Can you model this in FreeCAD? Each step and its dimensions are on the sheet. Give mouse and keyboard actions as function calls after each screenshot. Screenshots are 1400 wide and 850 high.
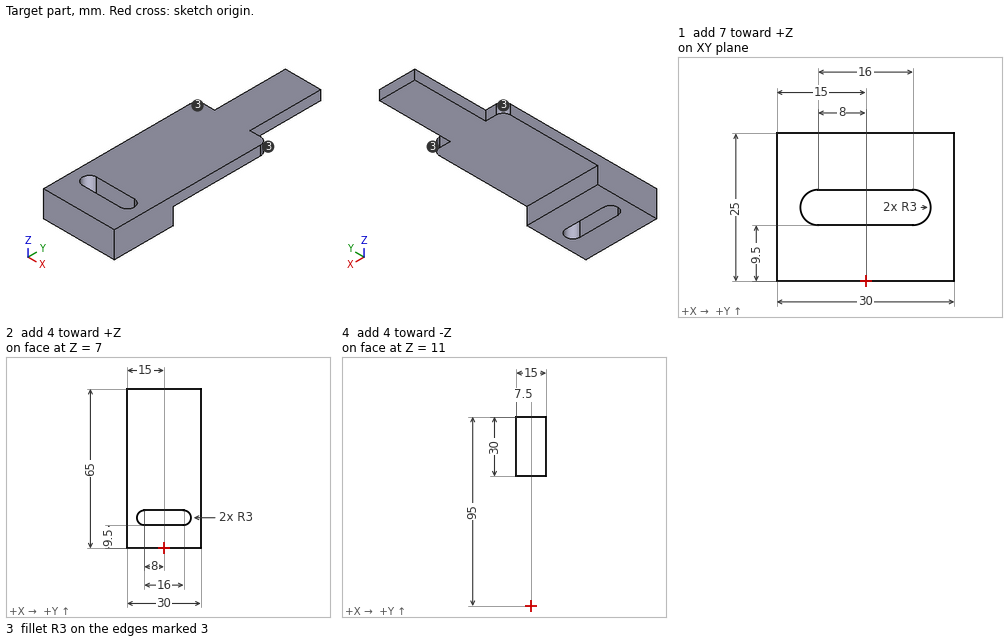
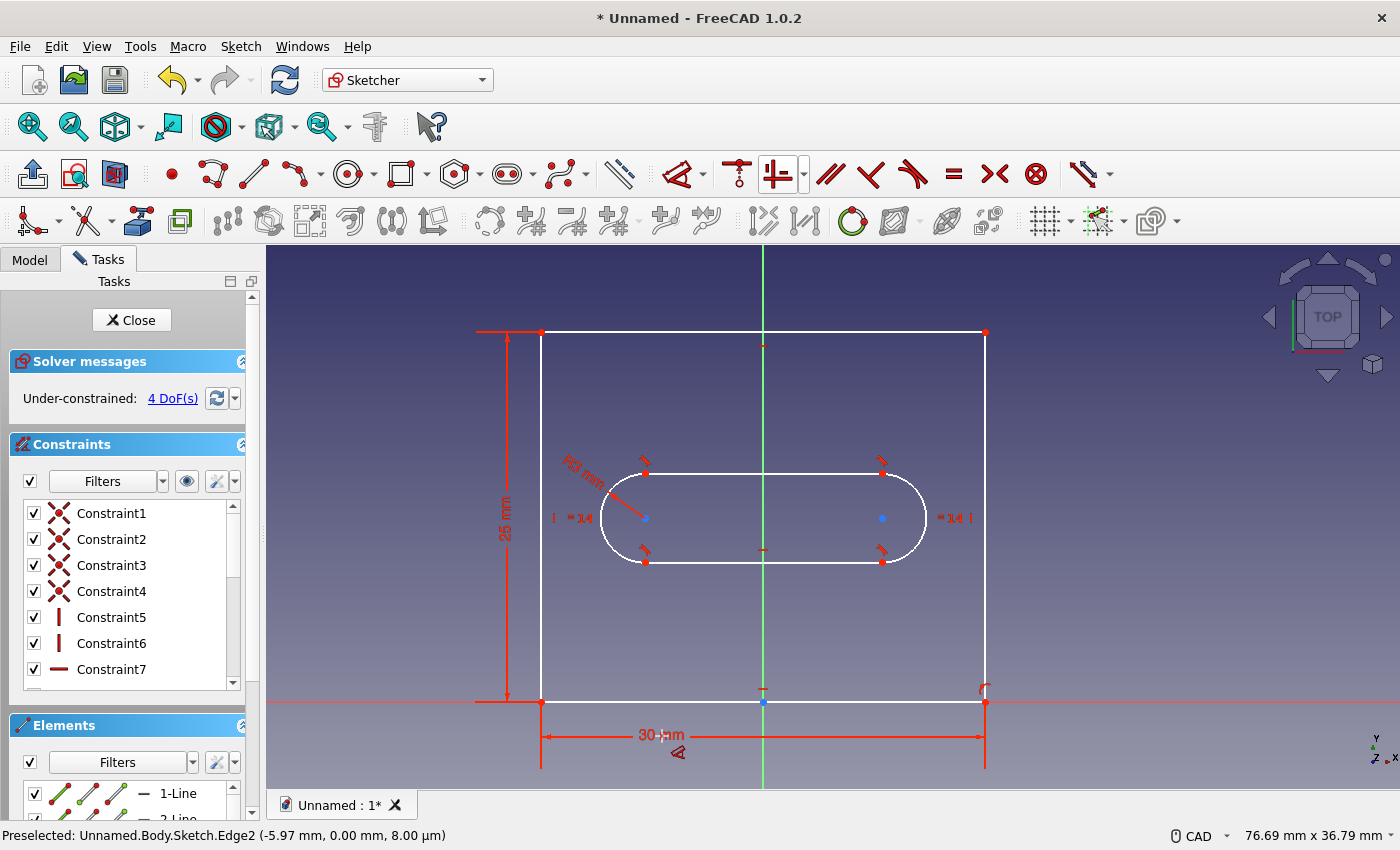
click(716, 474)
click(709, 440)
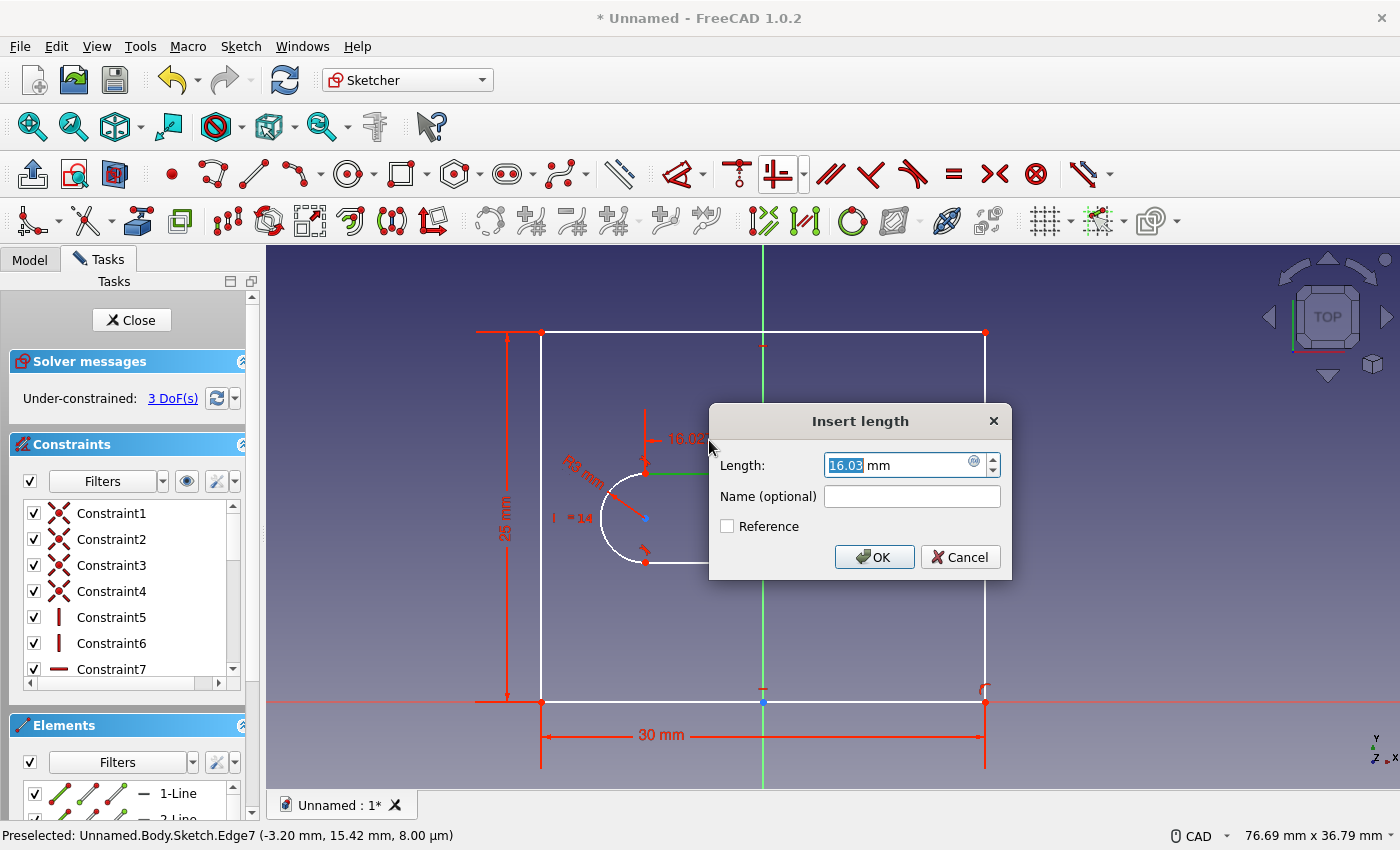
text(16)
key(Return)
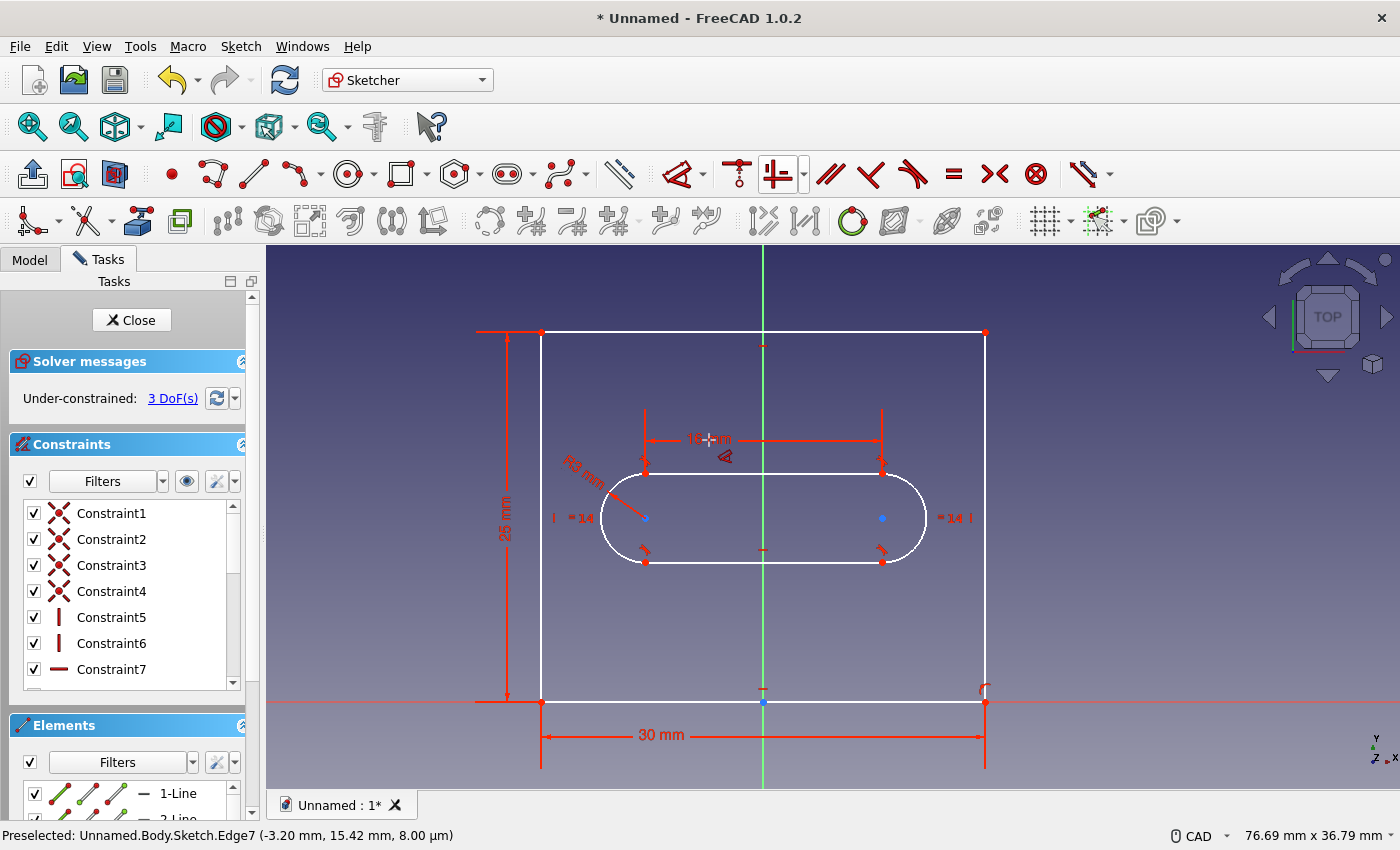
click(645, 474)
click(746, 736)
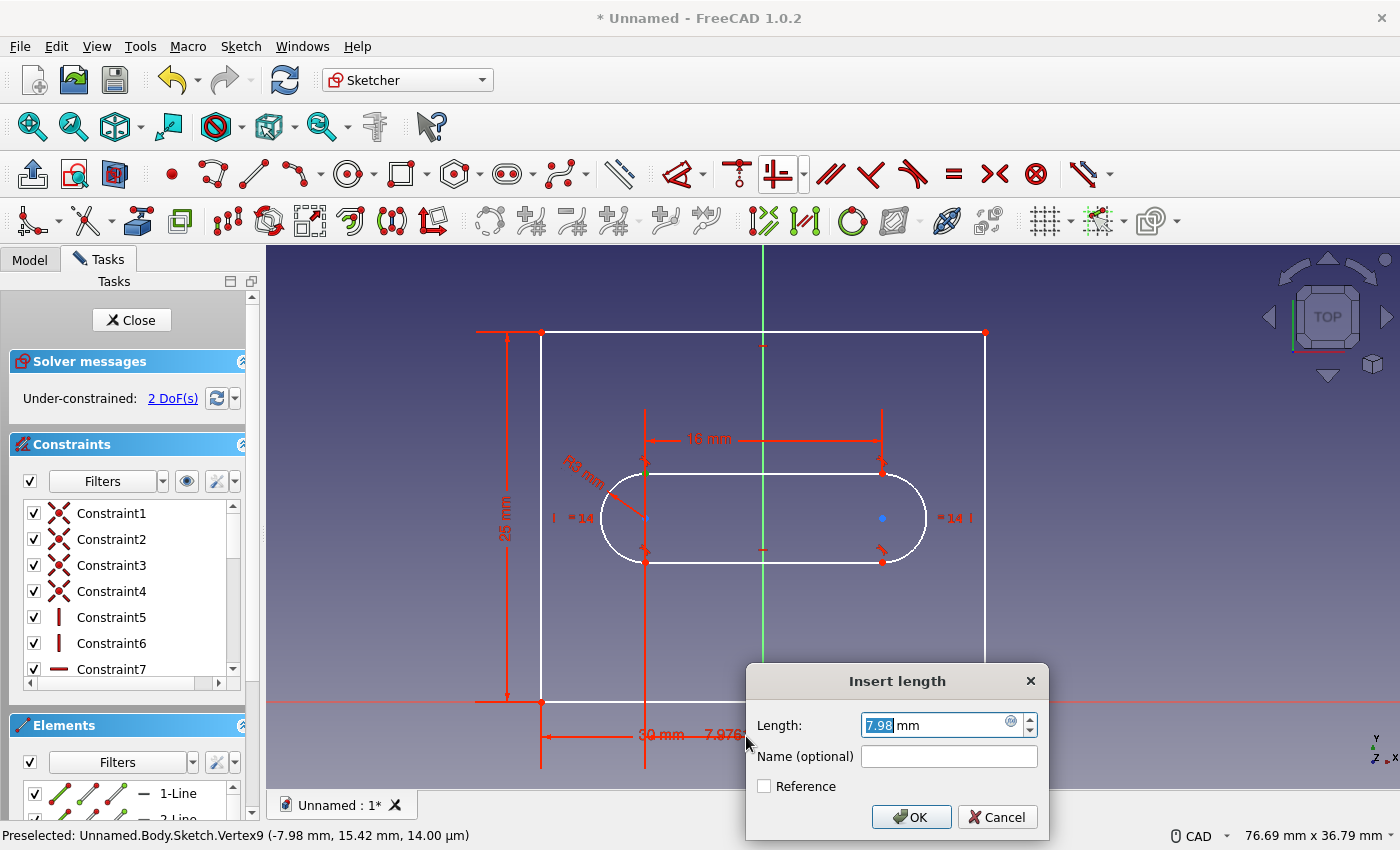
text(8)
key(Return)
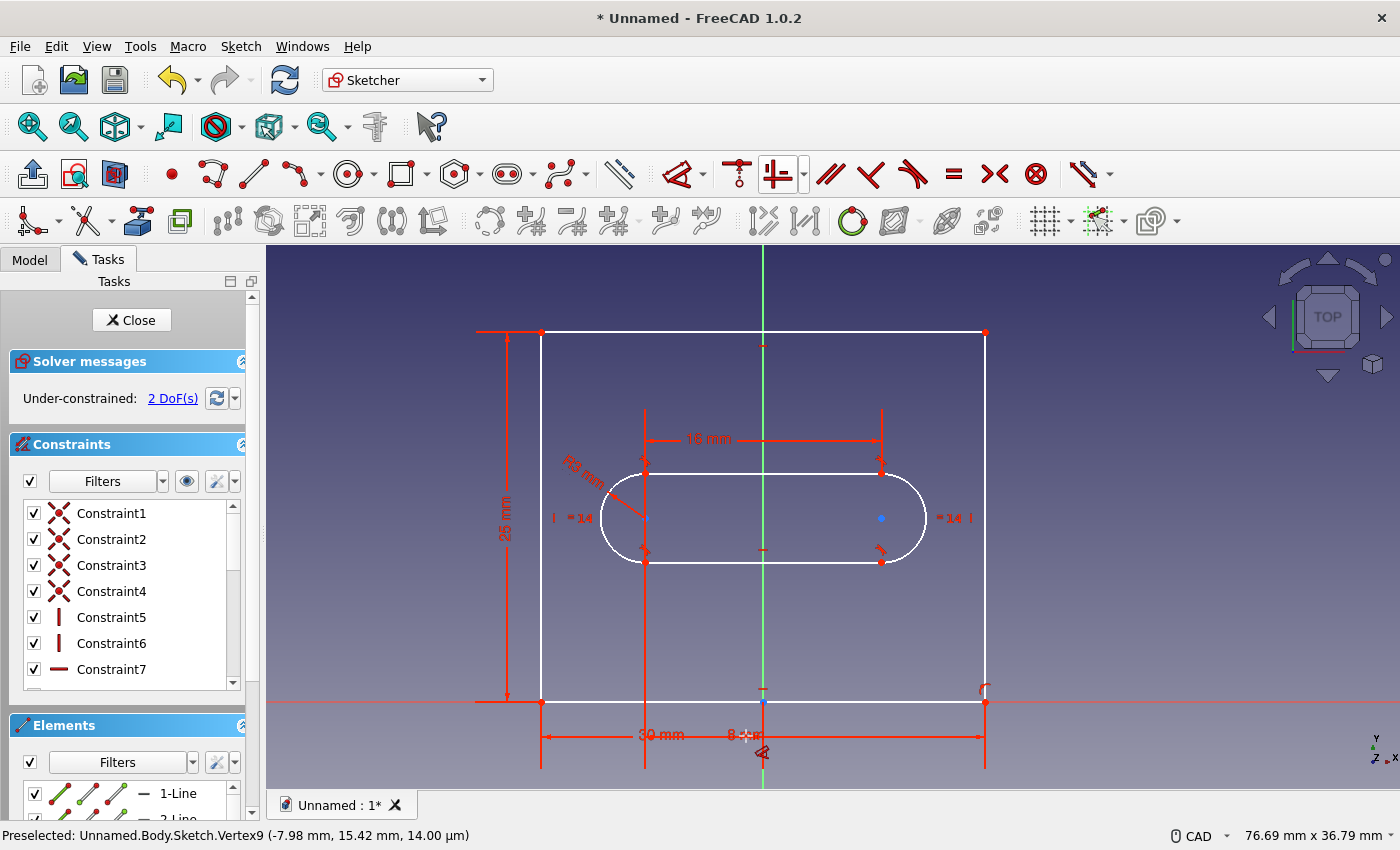
click(541, 332)
click(575, 736)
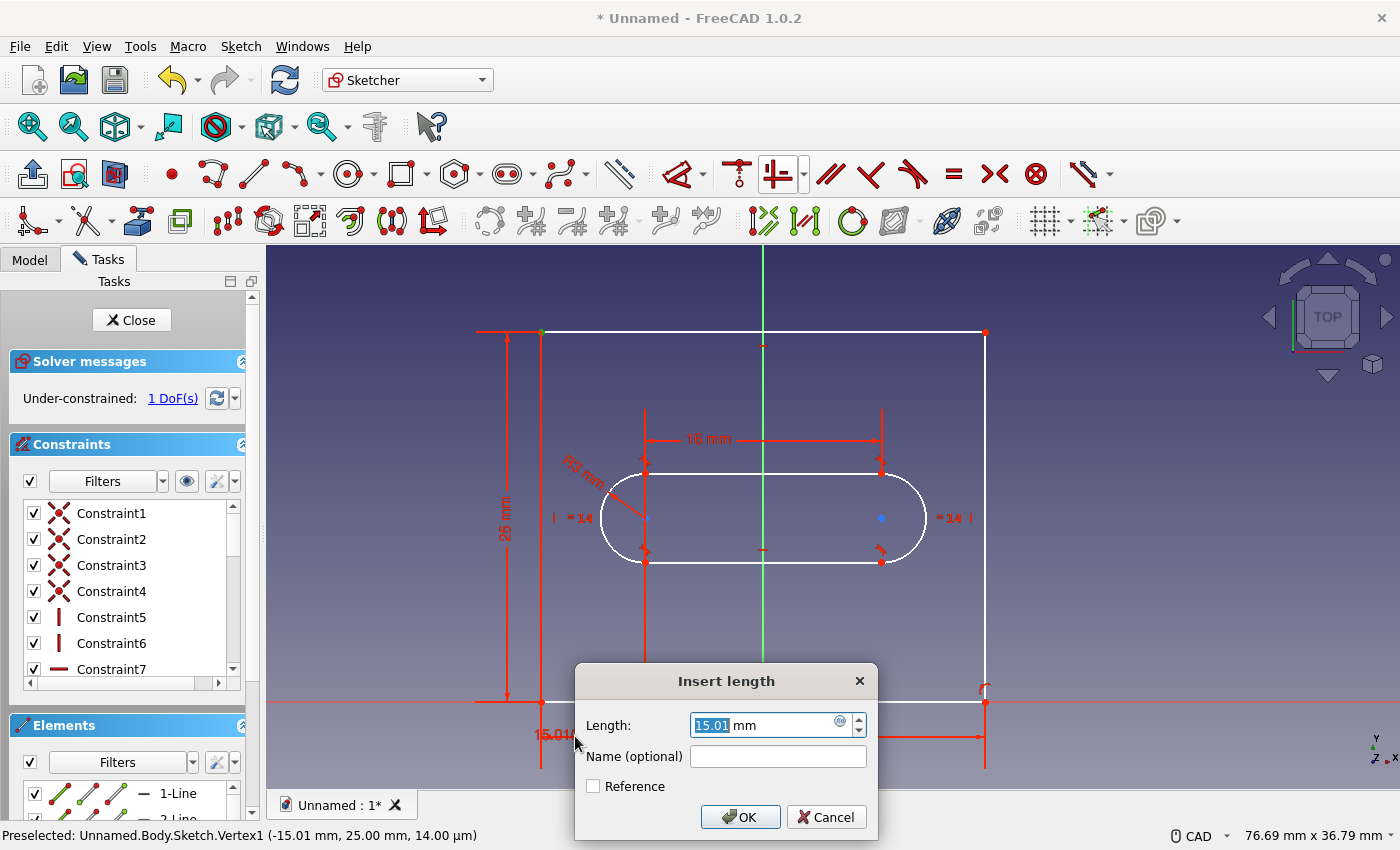
text(15)
key(Return)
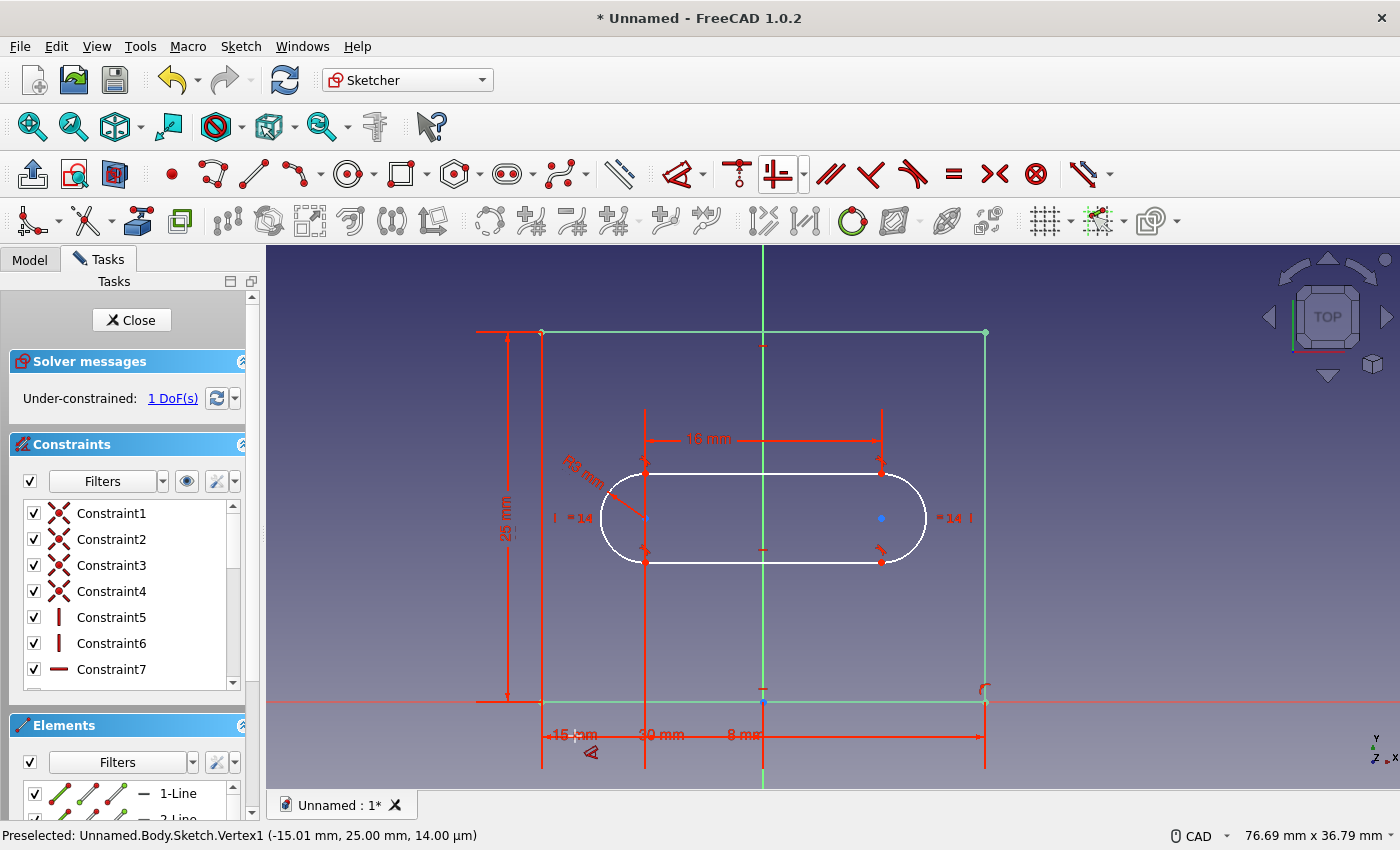
click(645, 563)
click(611, 632)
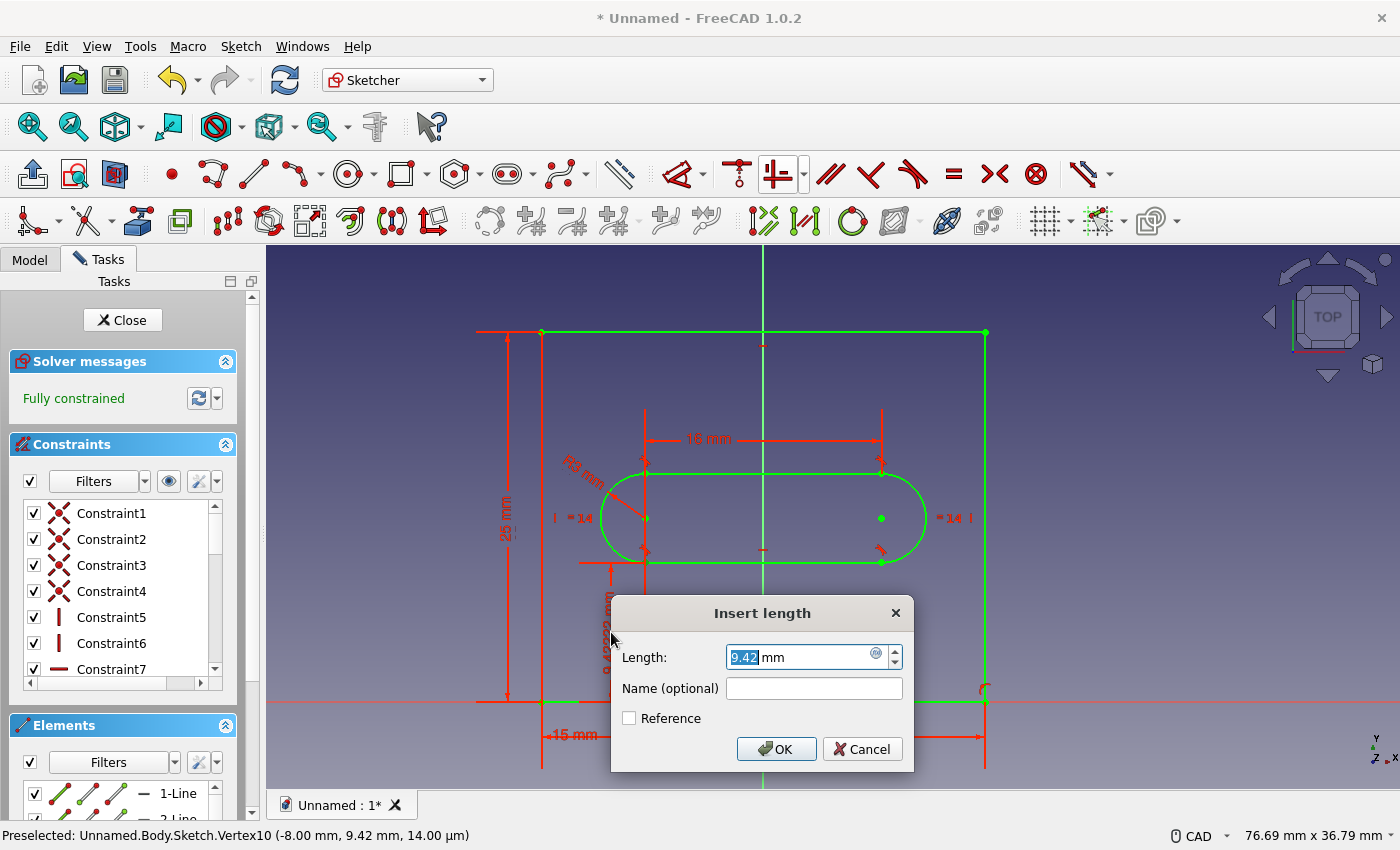
text(9.5)
key(Return)
key(Escape)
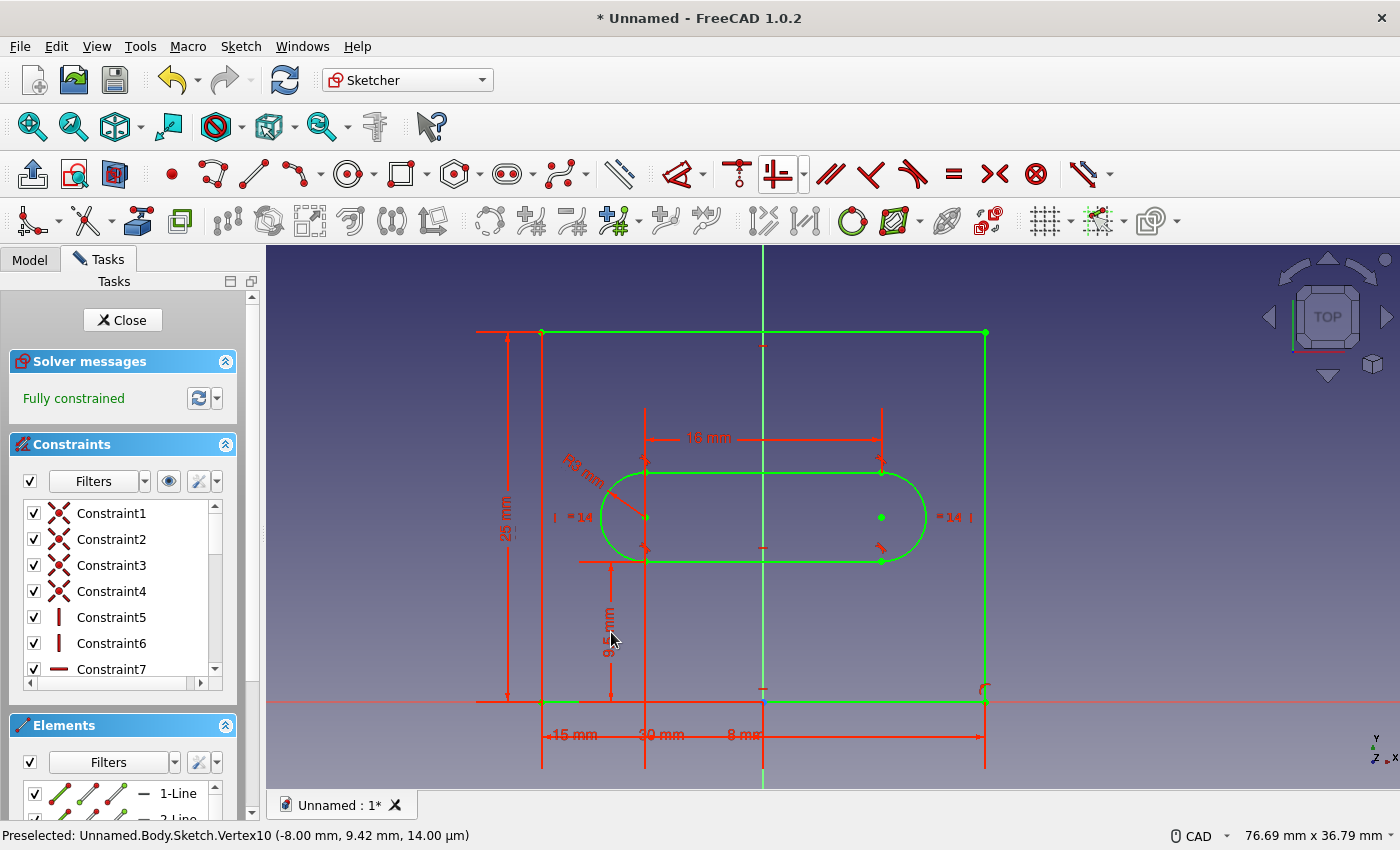
click(123, 320)